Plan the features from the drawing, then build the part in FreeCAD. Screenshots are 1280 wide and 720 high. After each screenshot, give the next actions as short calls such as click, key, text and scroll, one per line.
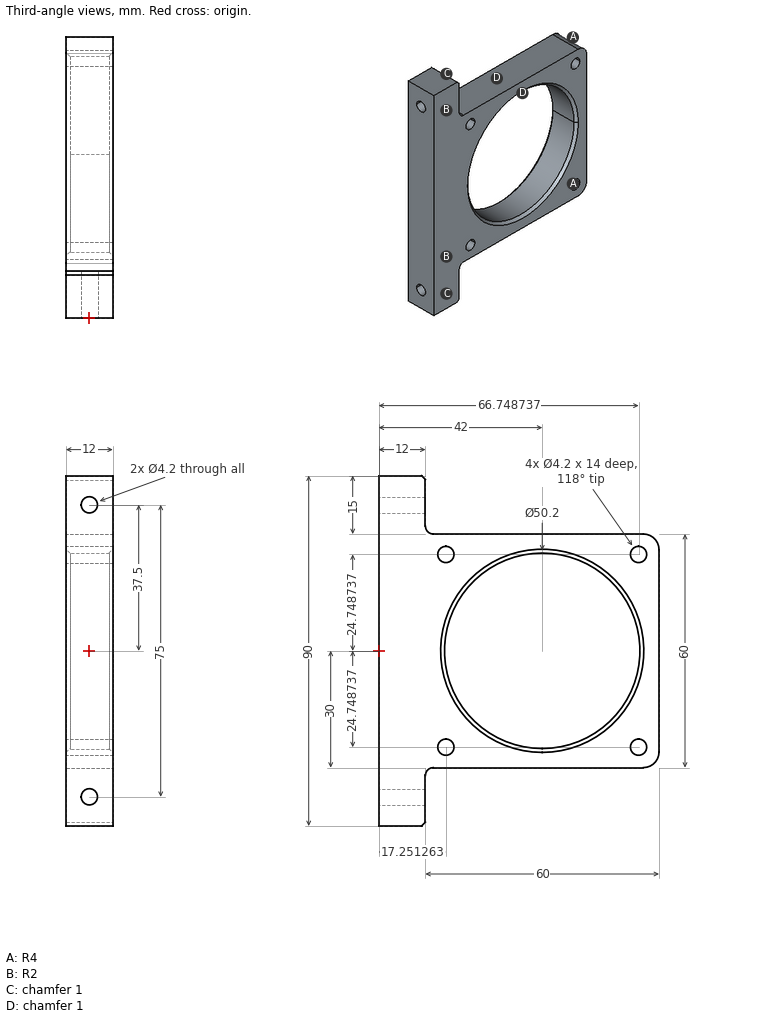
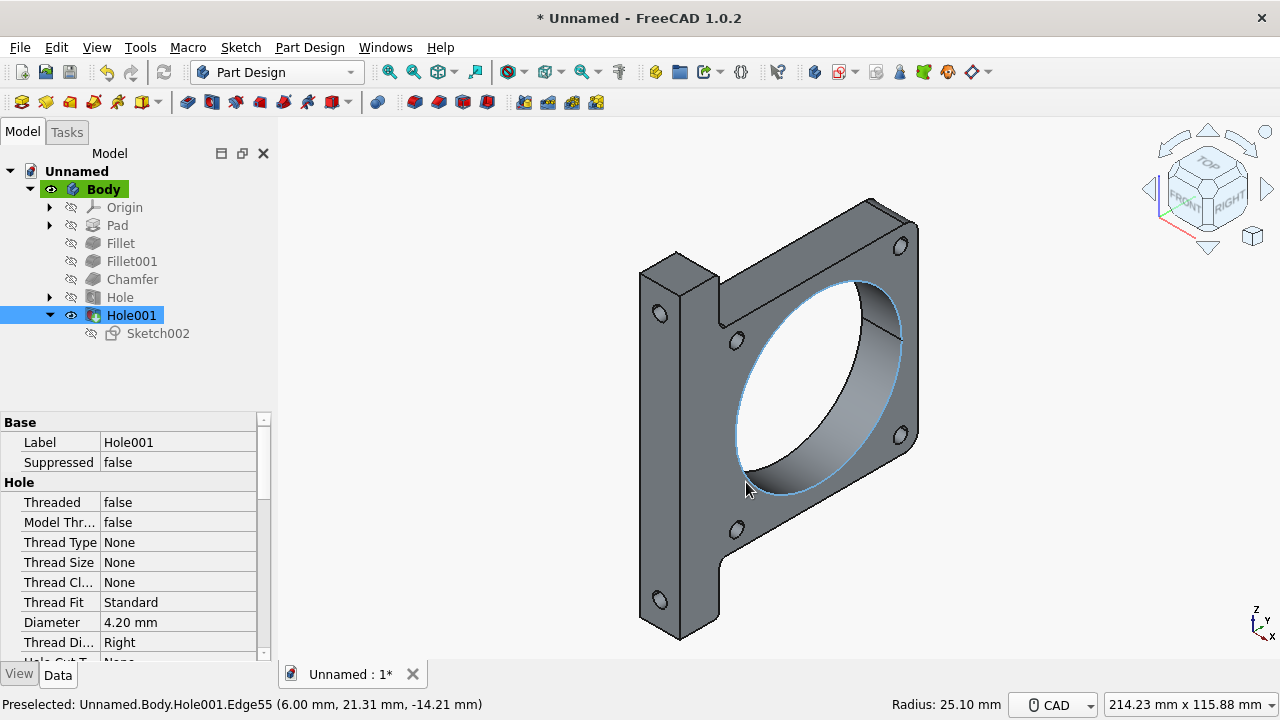
key(1)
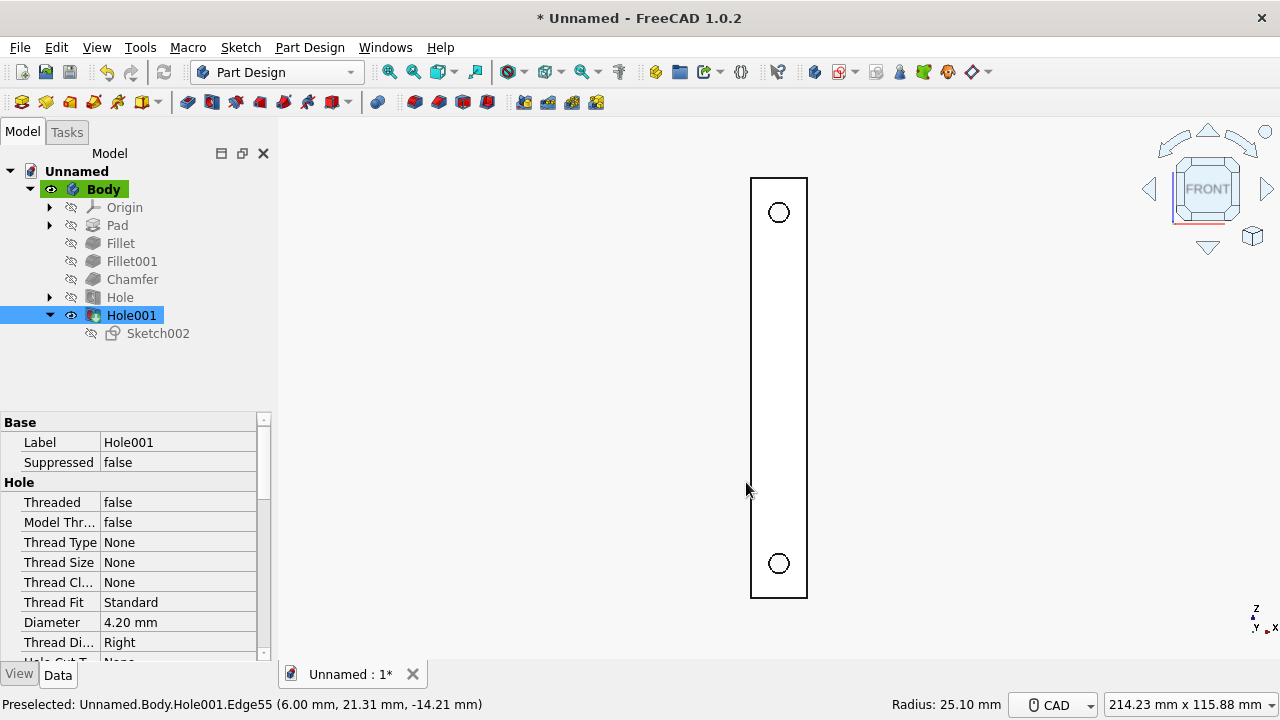
key(3)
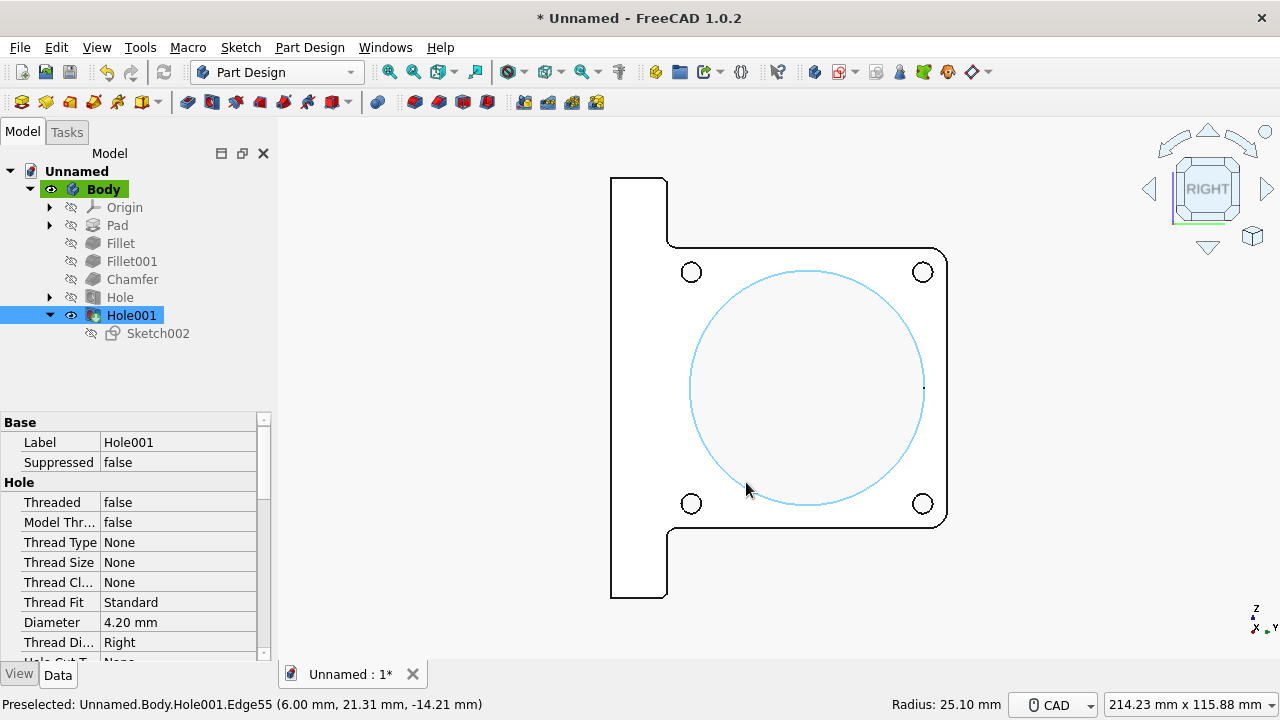
key(5)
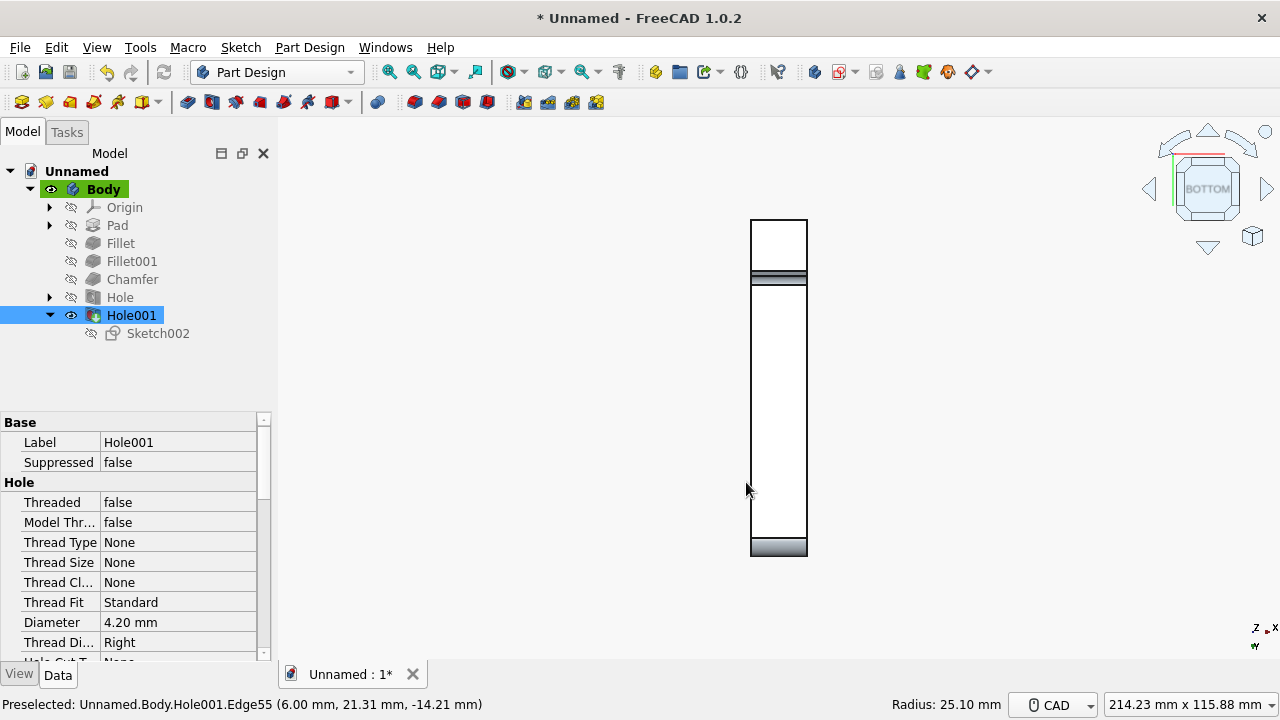
key(4)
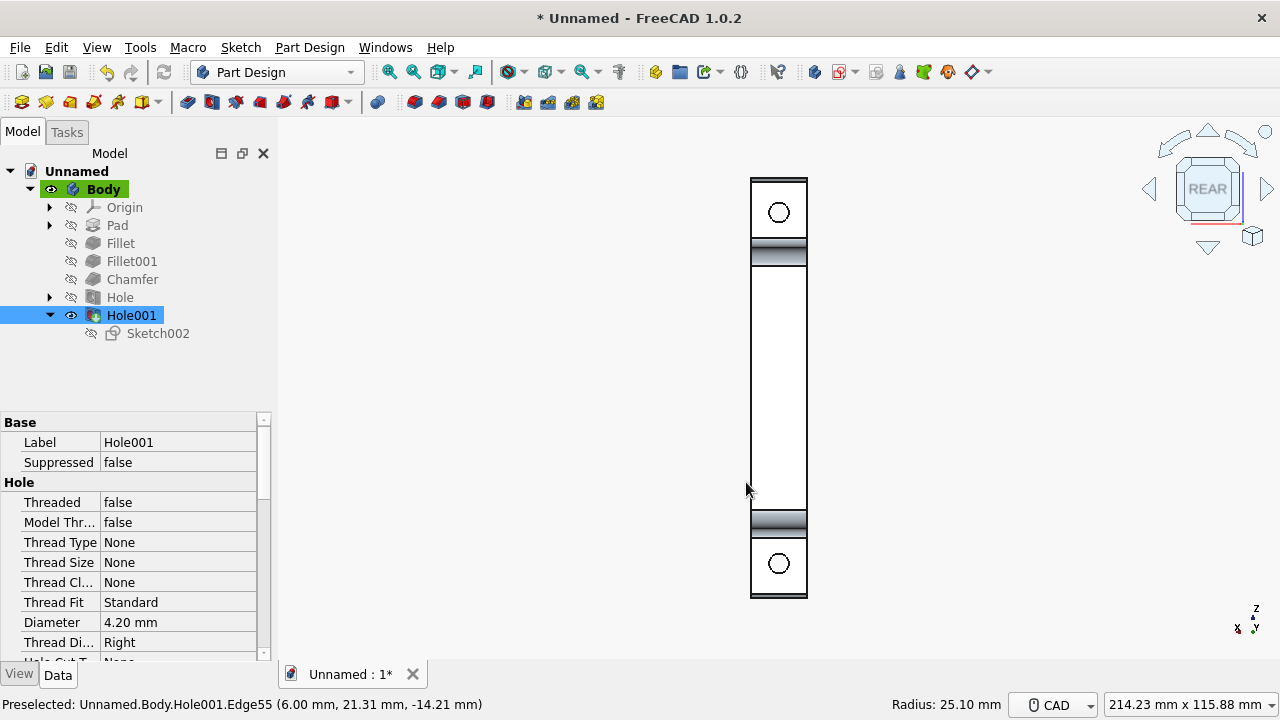
key(6)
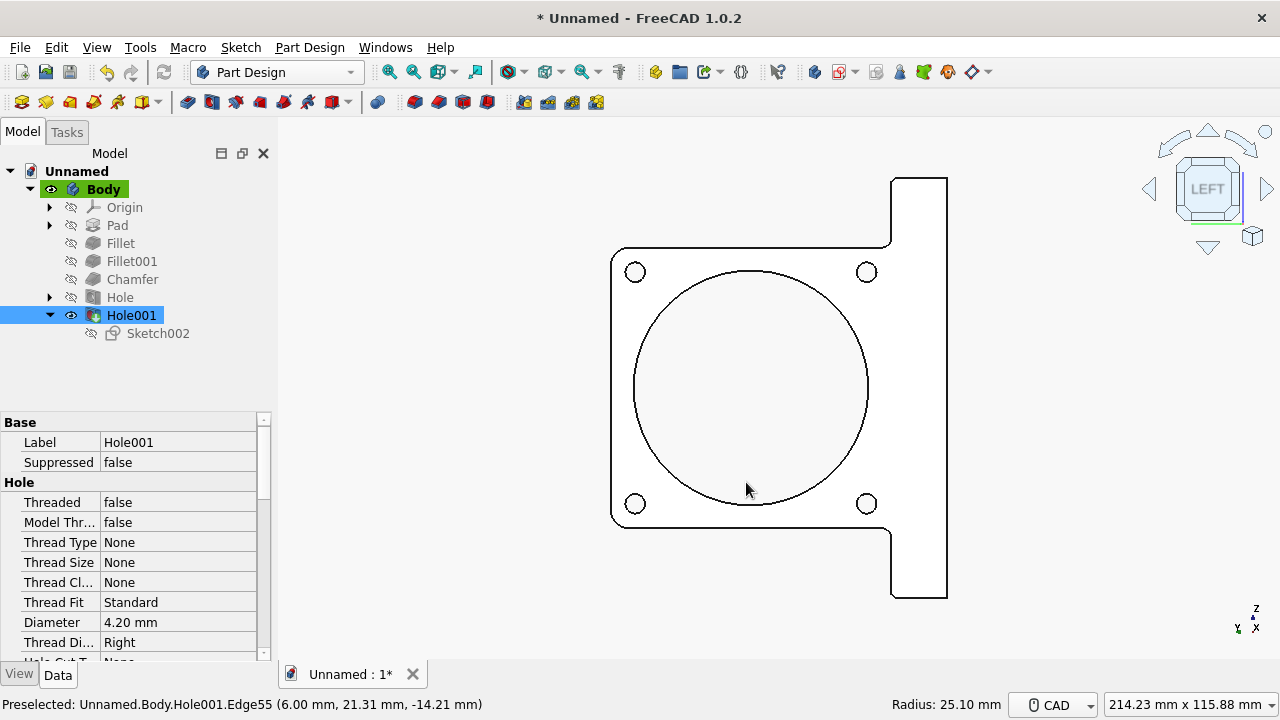
click(868, 387, ctrl)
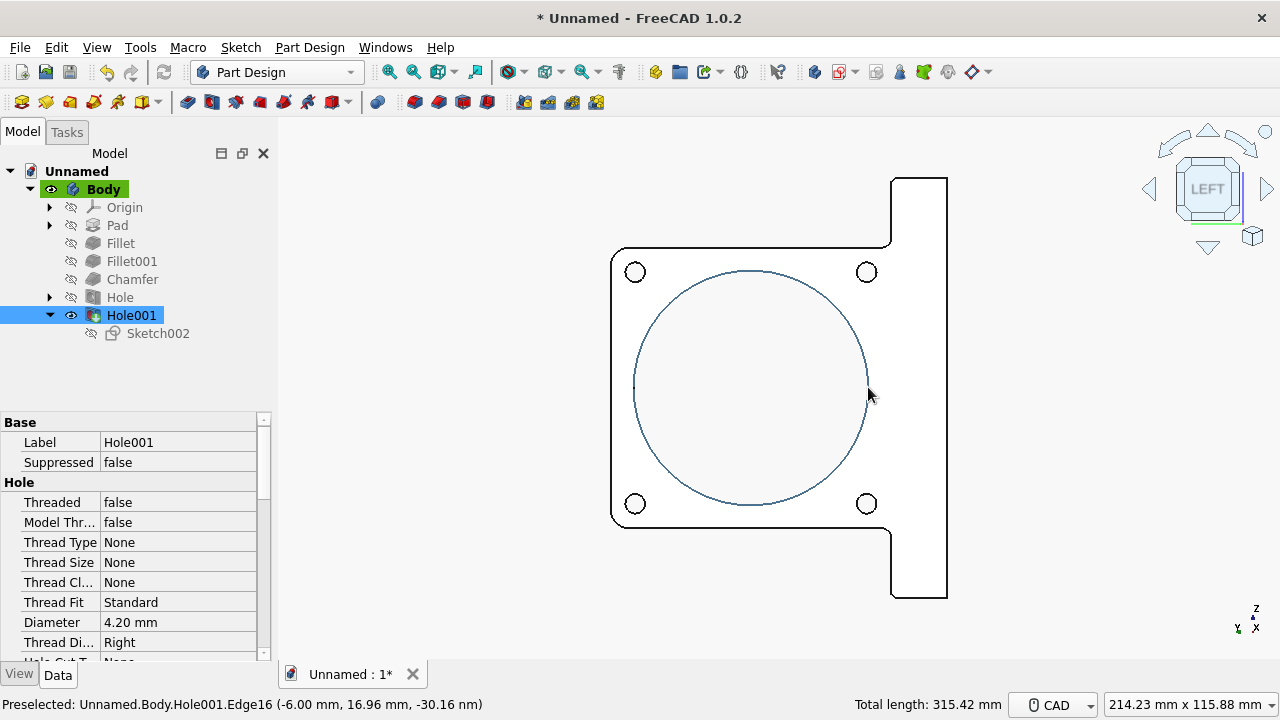
click(440, 102)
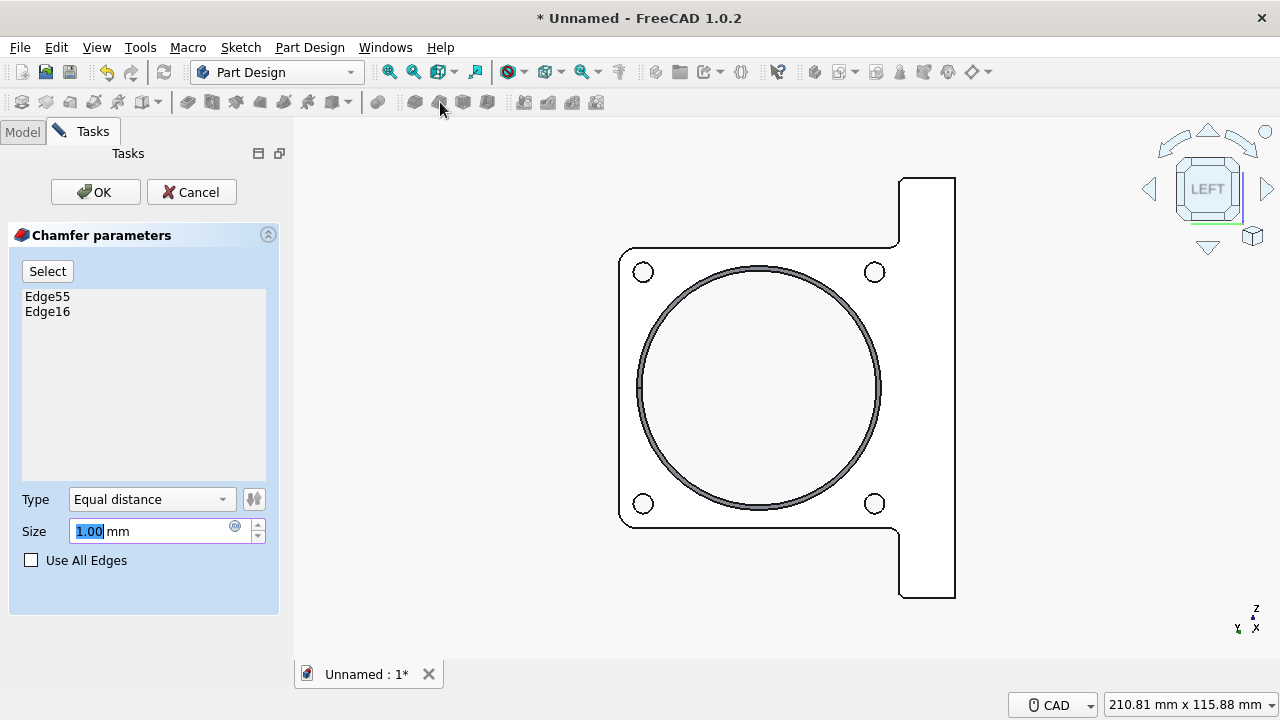
text(1)
key(Tab)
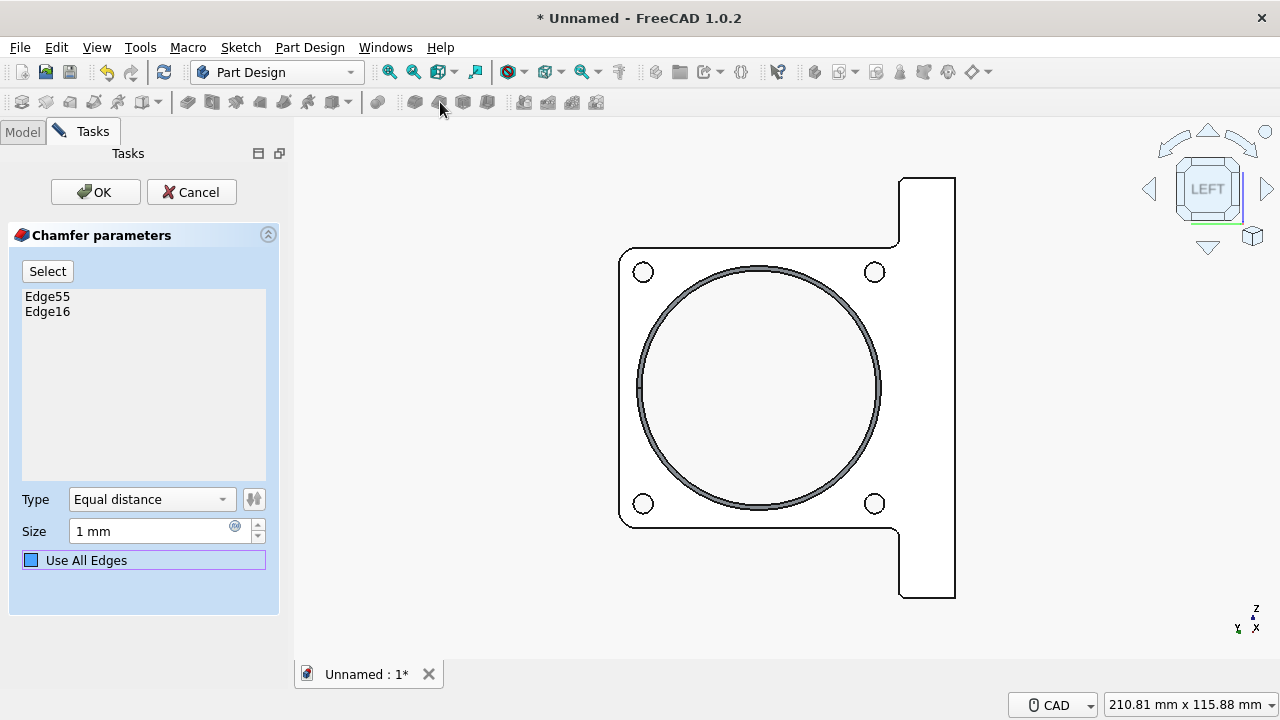
click(96, 192)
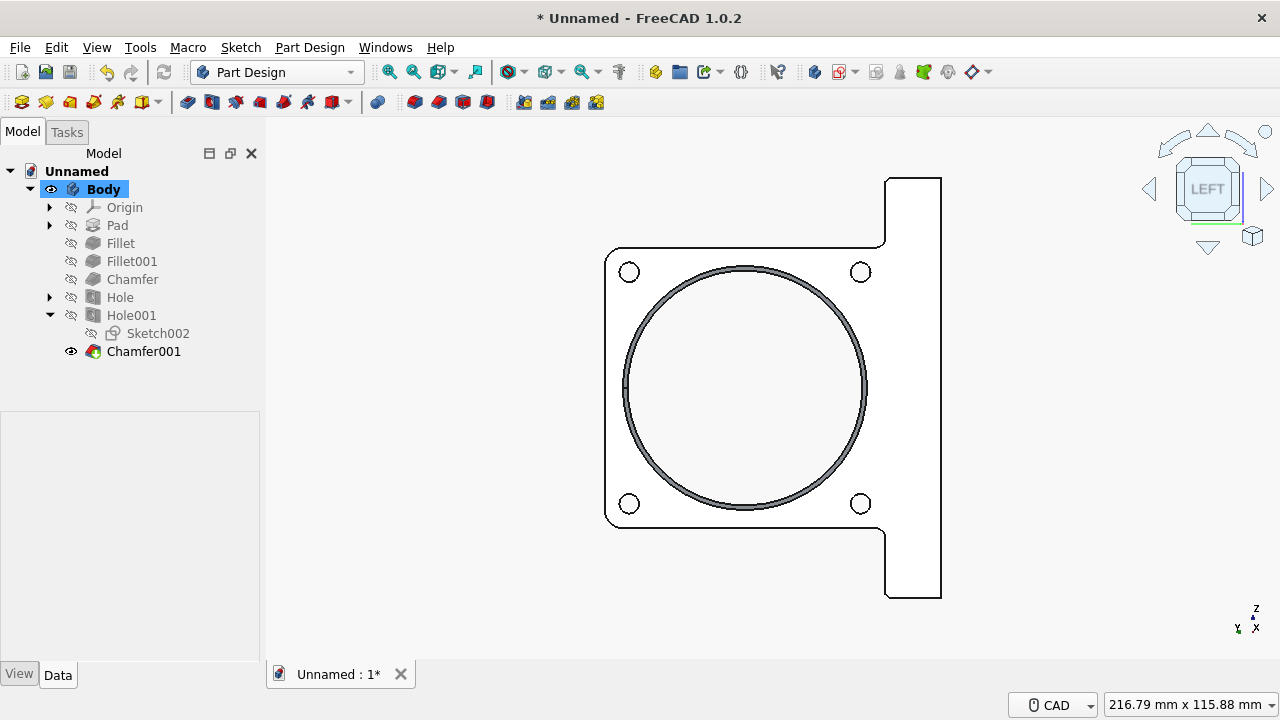
key(0)